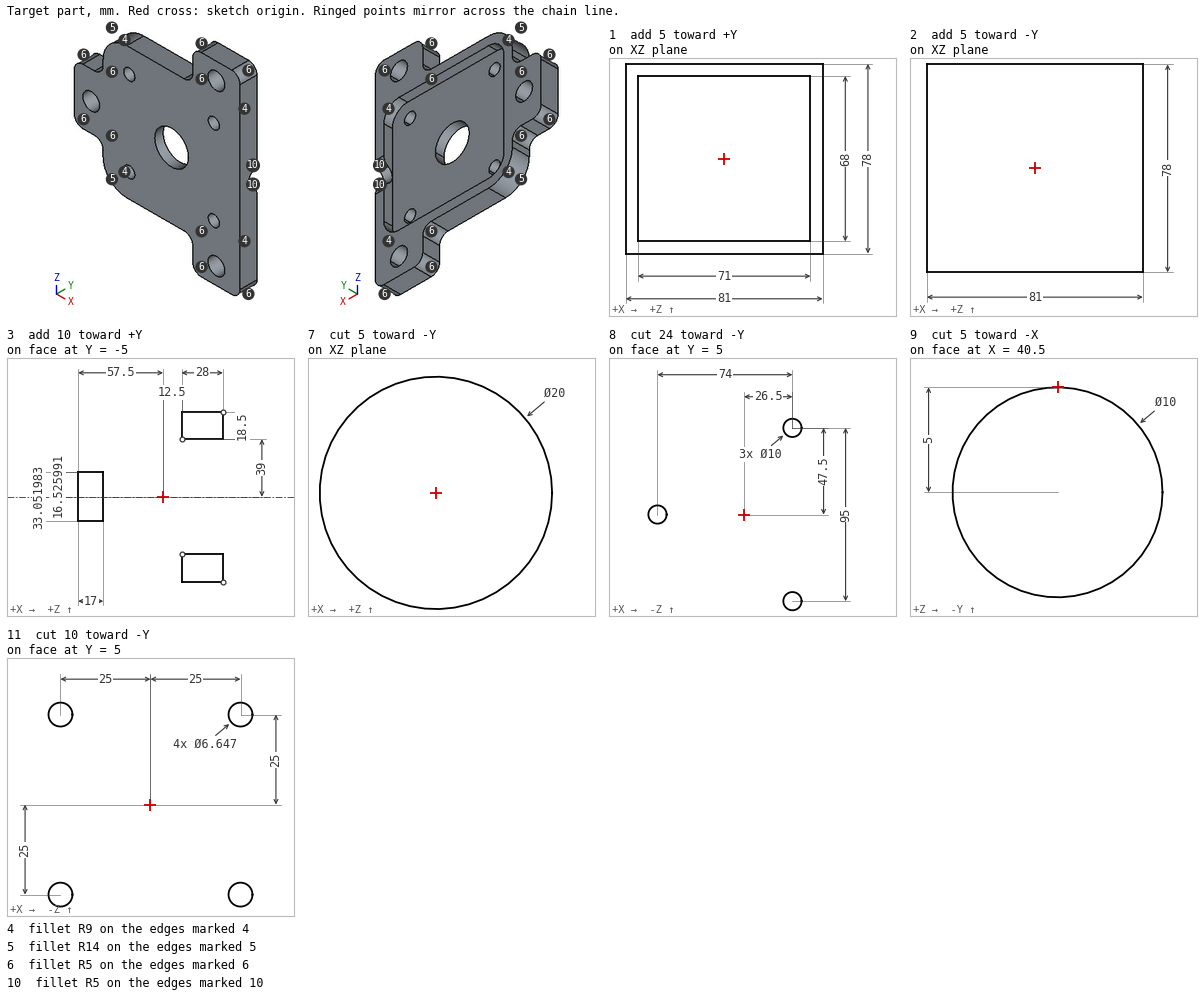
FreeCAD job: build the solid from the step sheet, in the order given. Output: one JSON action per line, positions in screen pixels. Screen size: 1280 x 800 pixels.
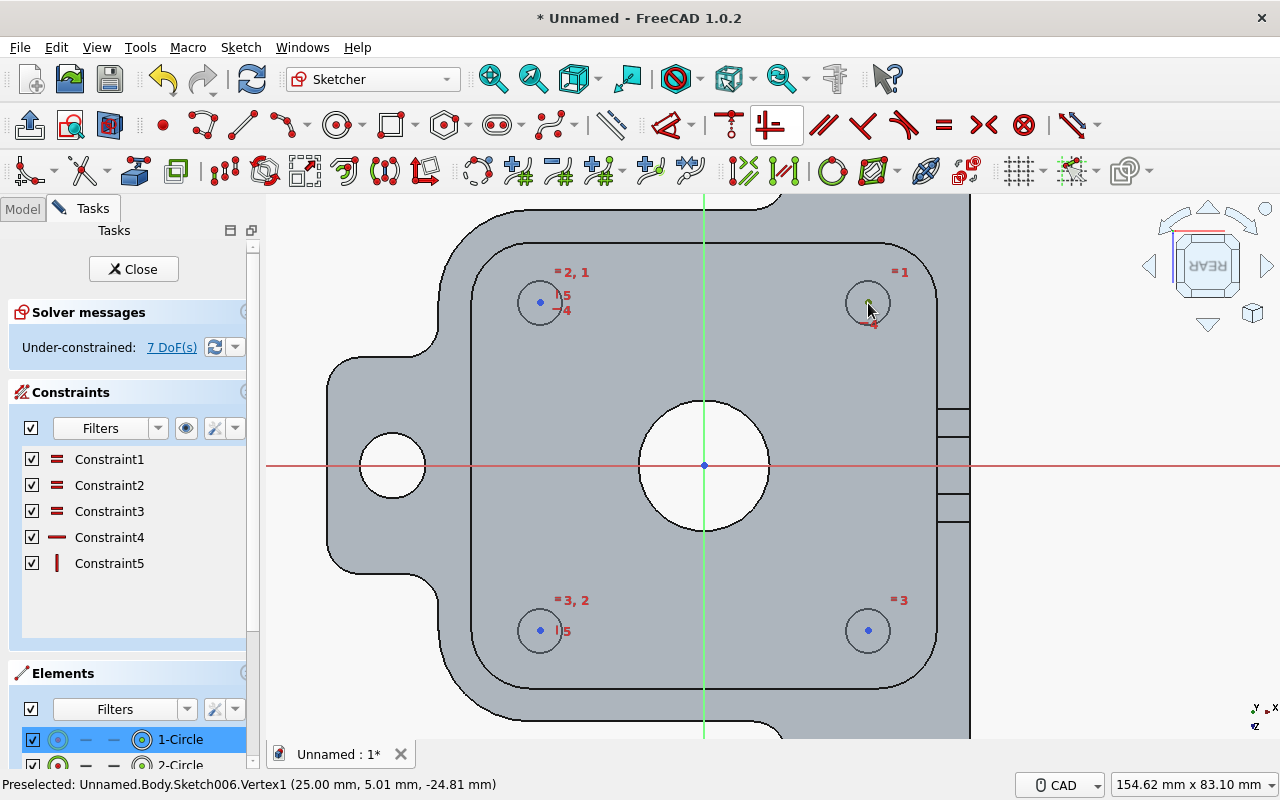
{"action": "left_click", "coordinate": [868, 631]}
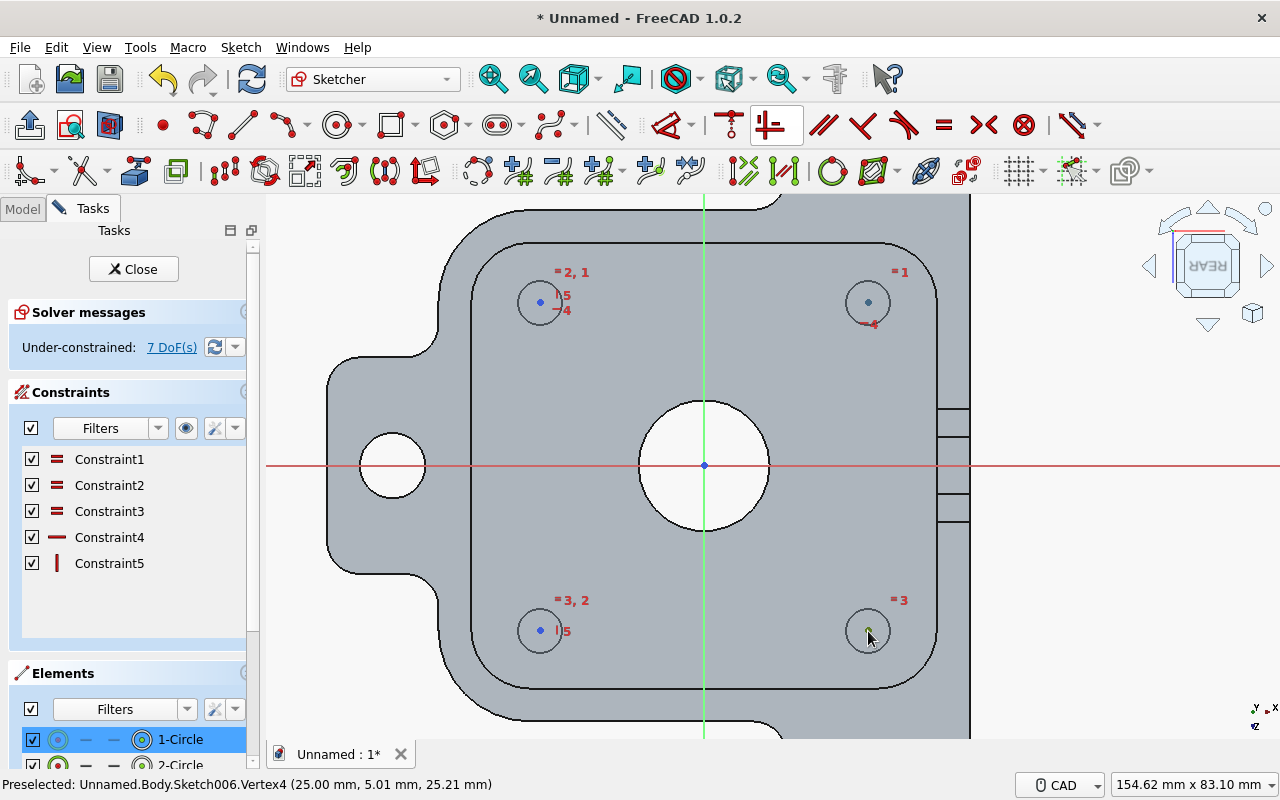
{"action": "left_click", "coordinate": [798, 126]}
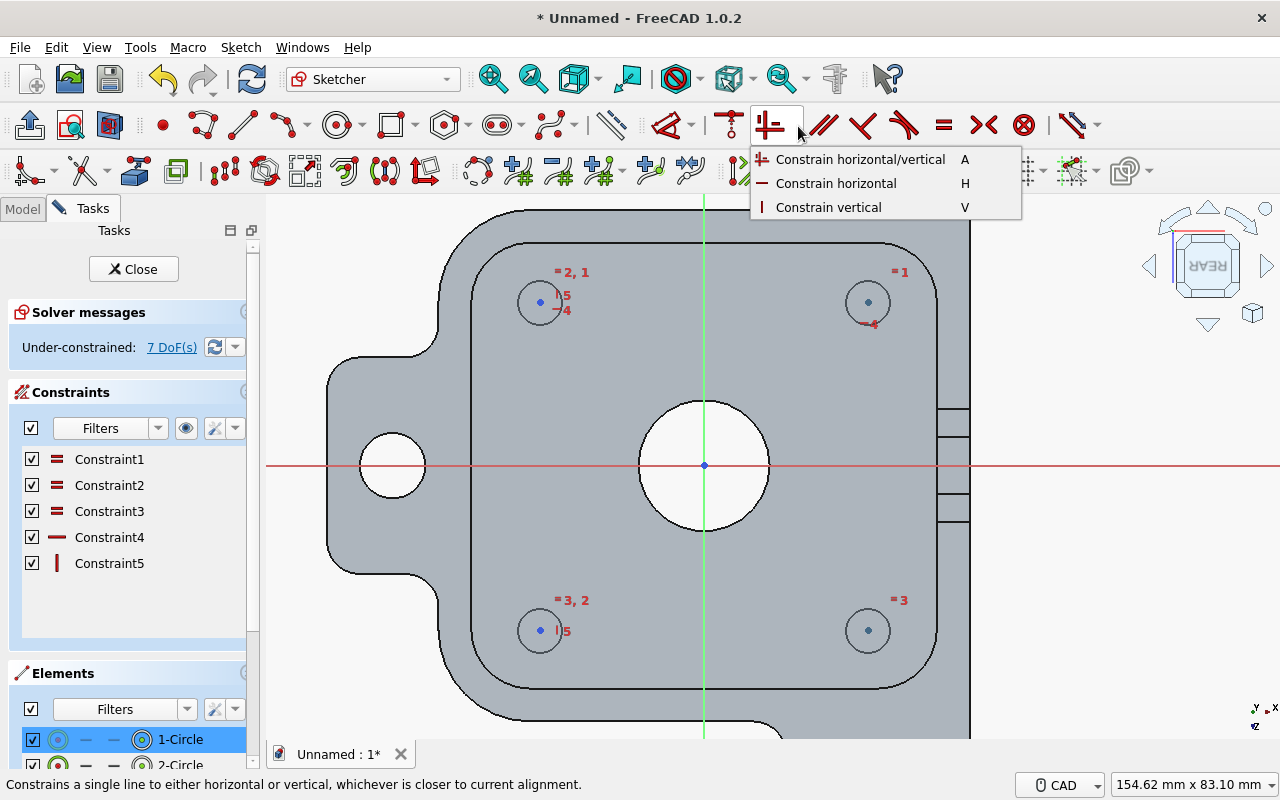
{"action": "left_click", "coordinate": [886, 207]}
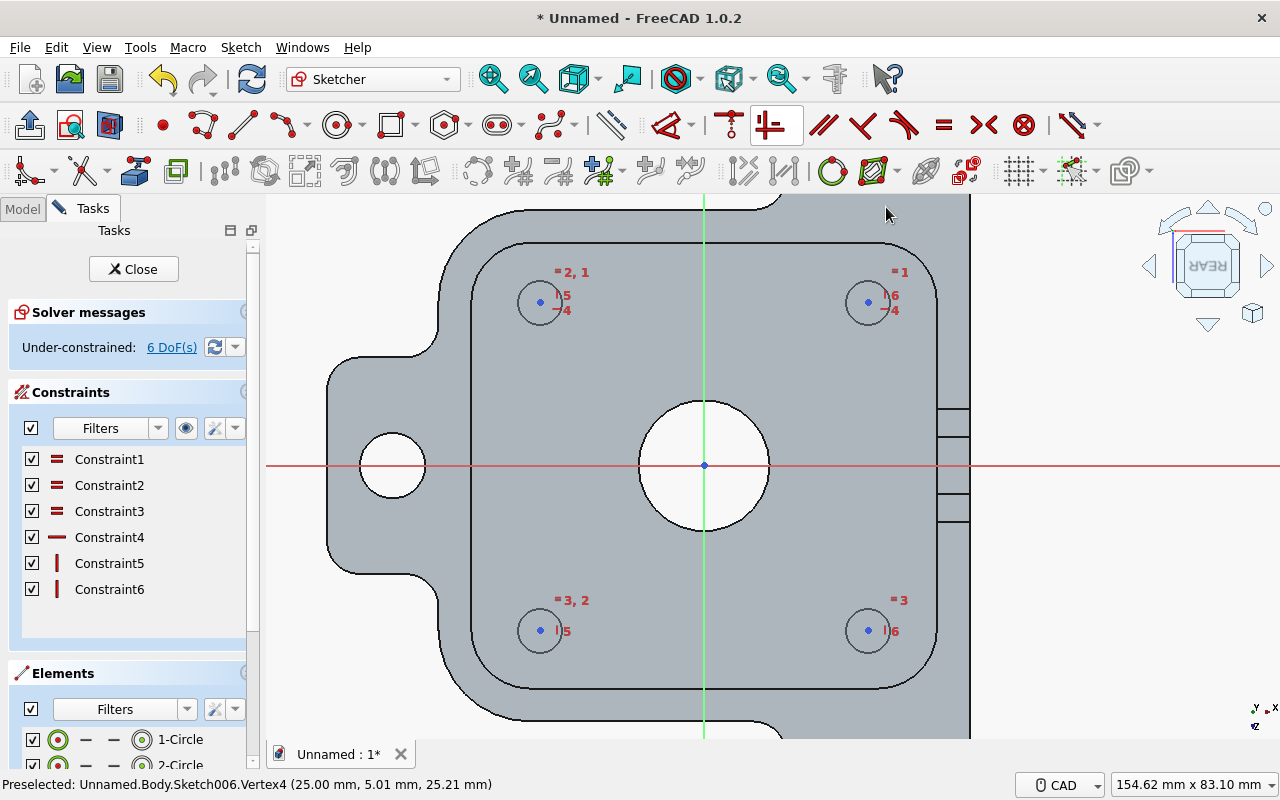
{"action": "left_click", "coordinate": [540, 631]}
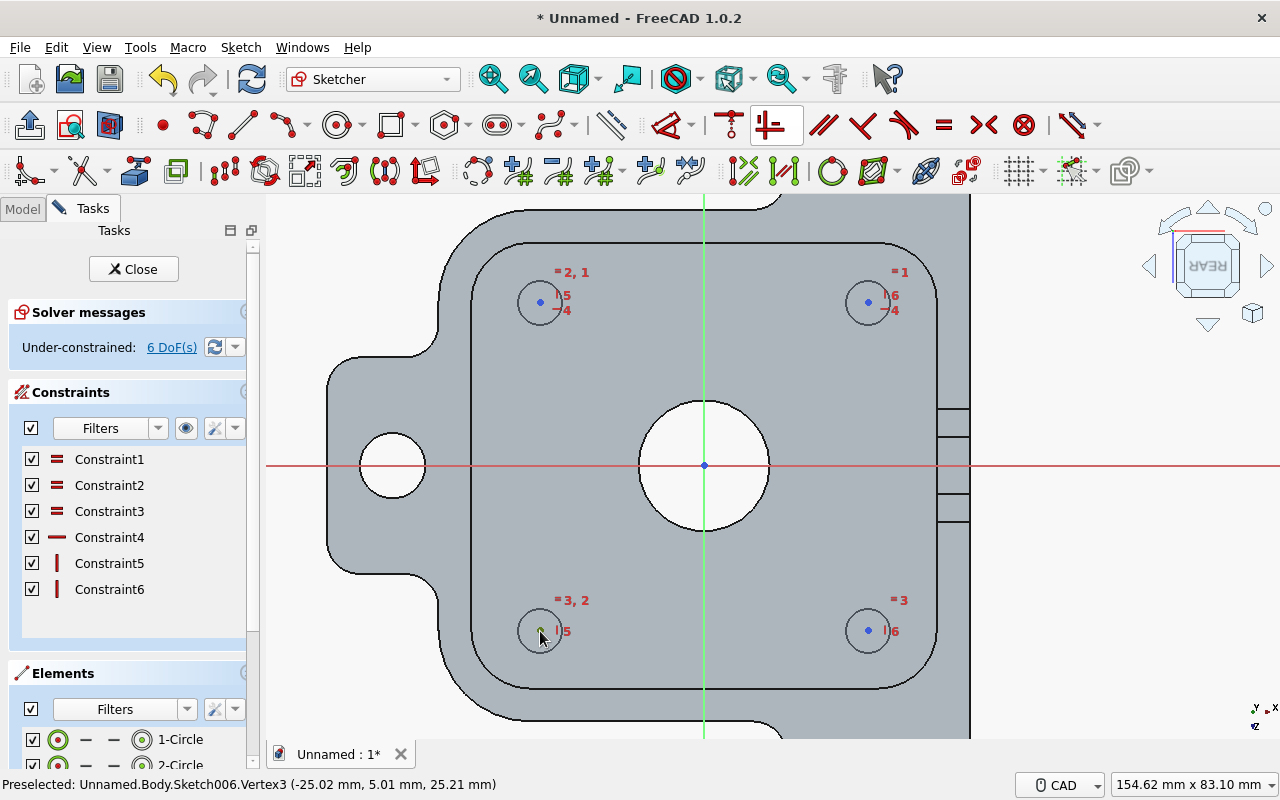
{"action": "left_click", "coordinate": [868, 631]}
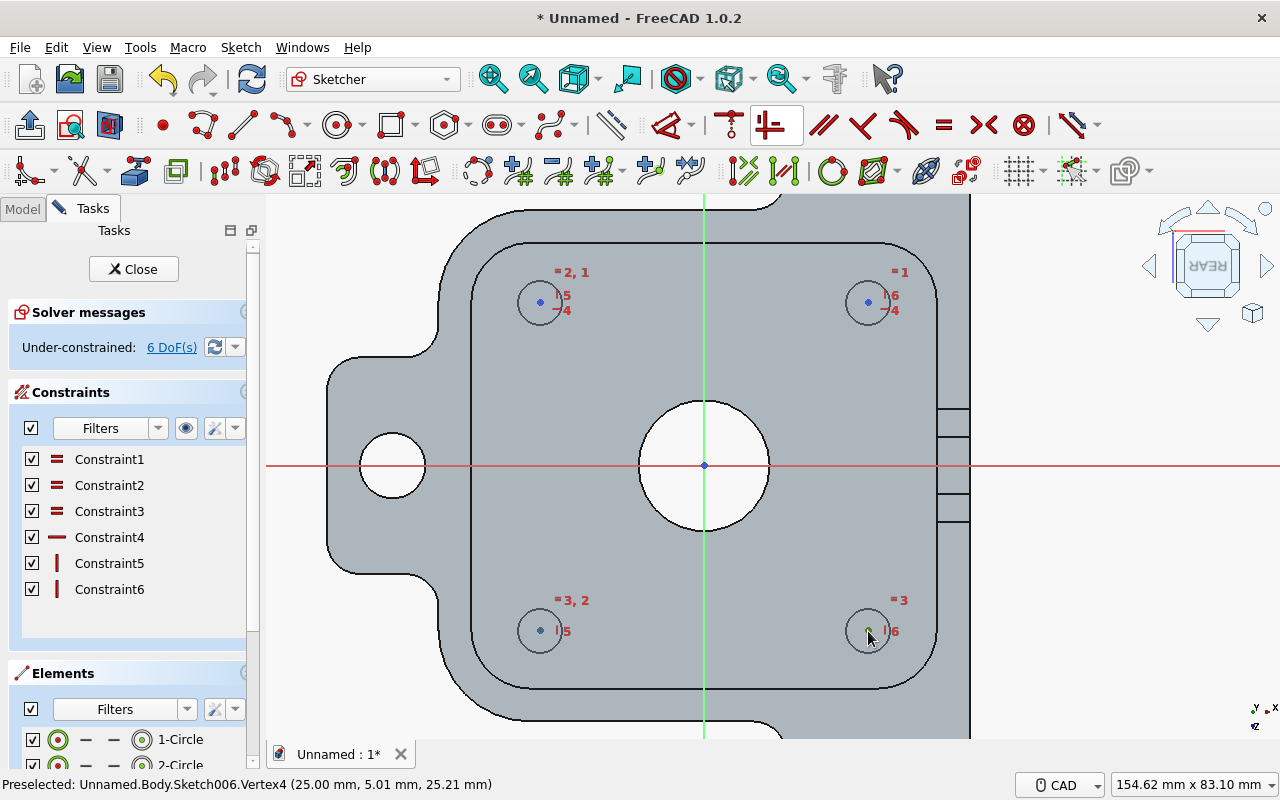
{"action": "key", "text": "h"}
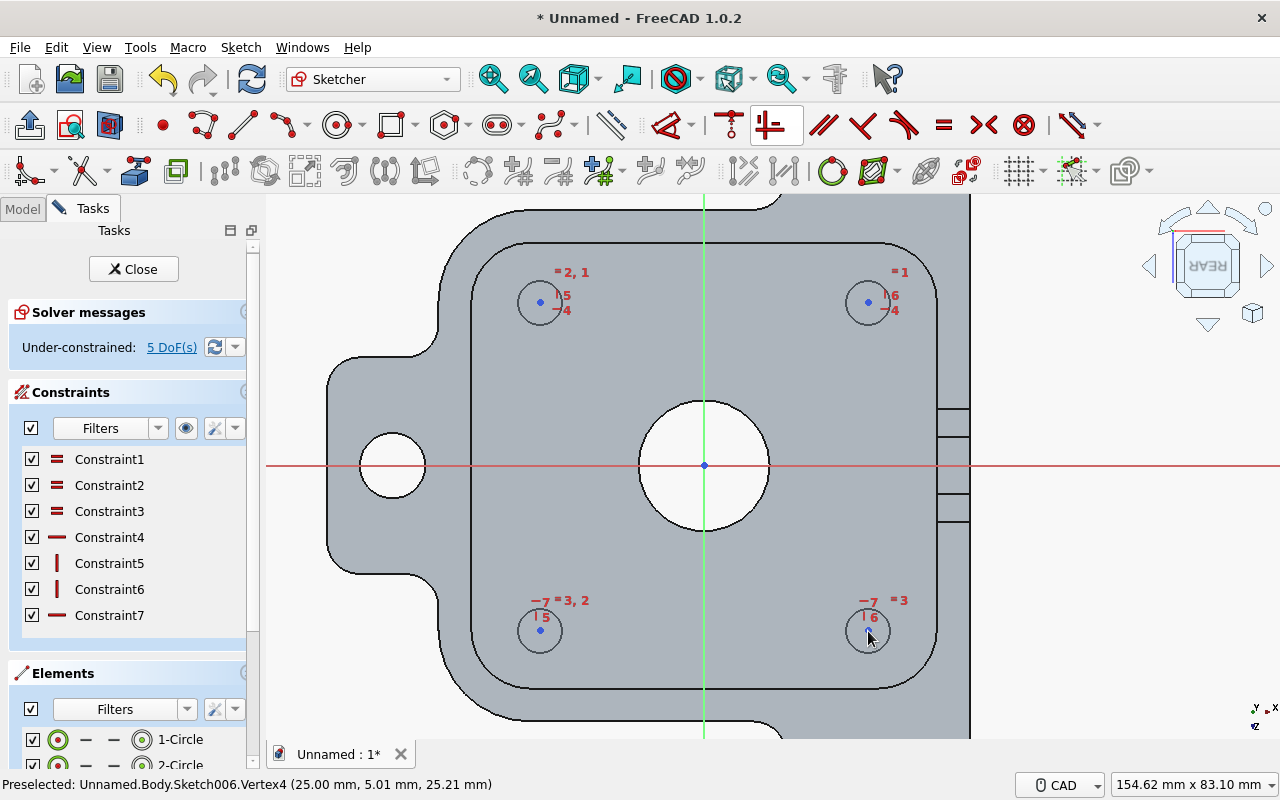
{"action": "key", "text": "d"}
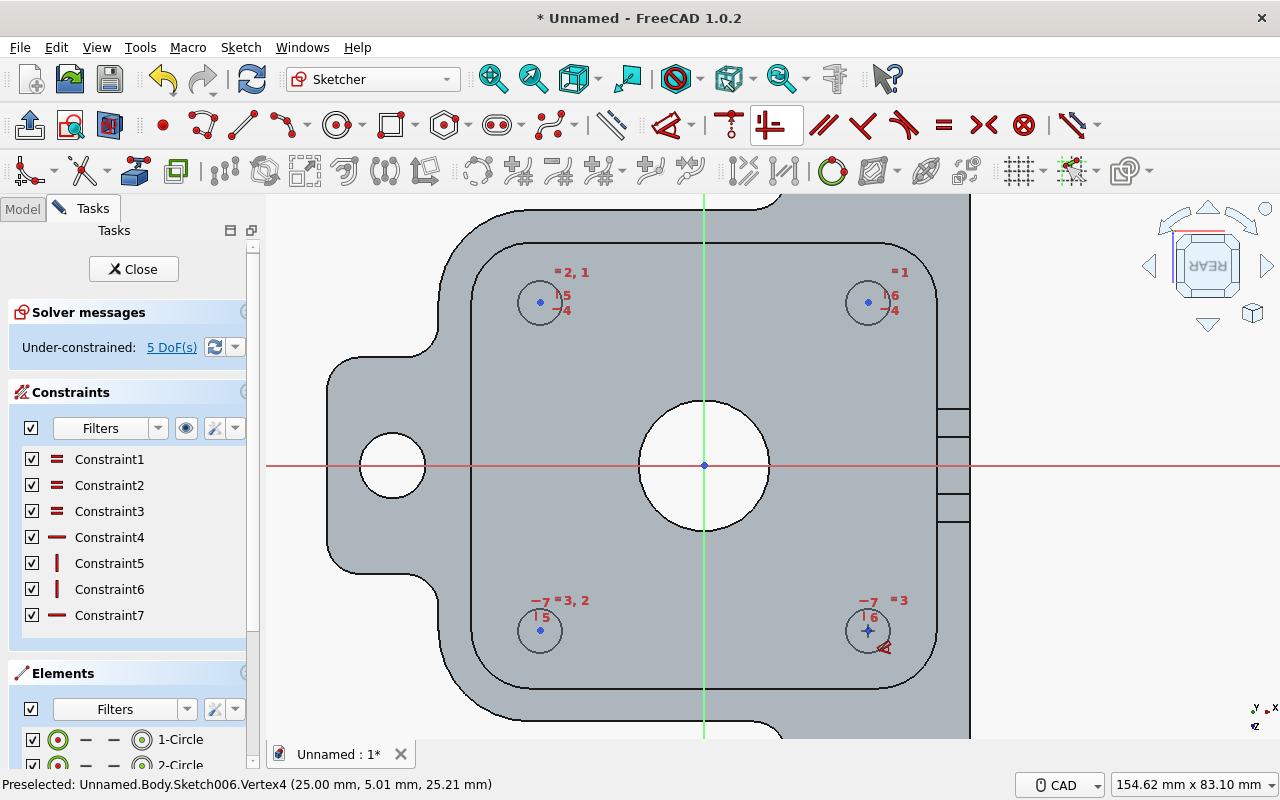
{"action": "left_click", "coordinate": [883, 287]}
{"action": "left_click", "coordinate": [905, 264]}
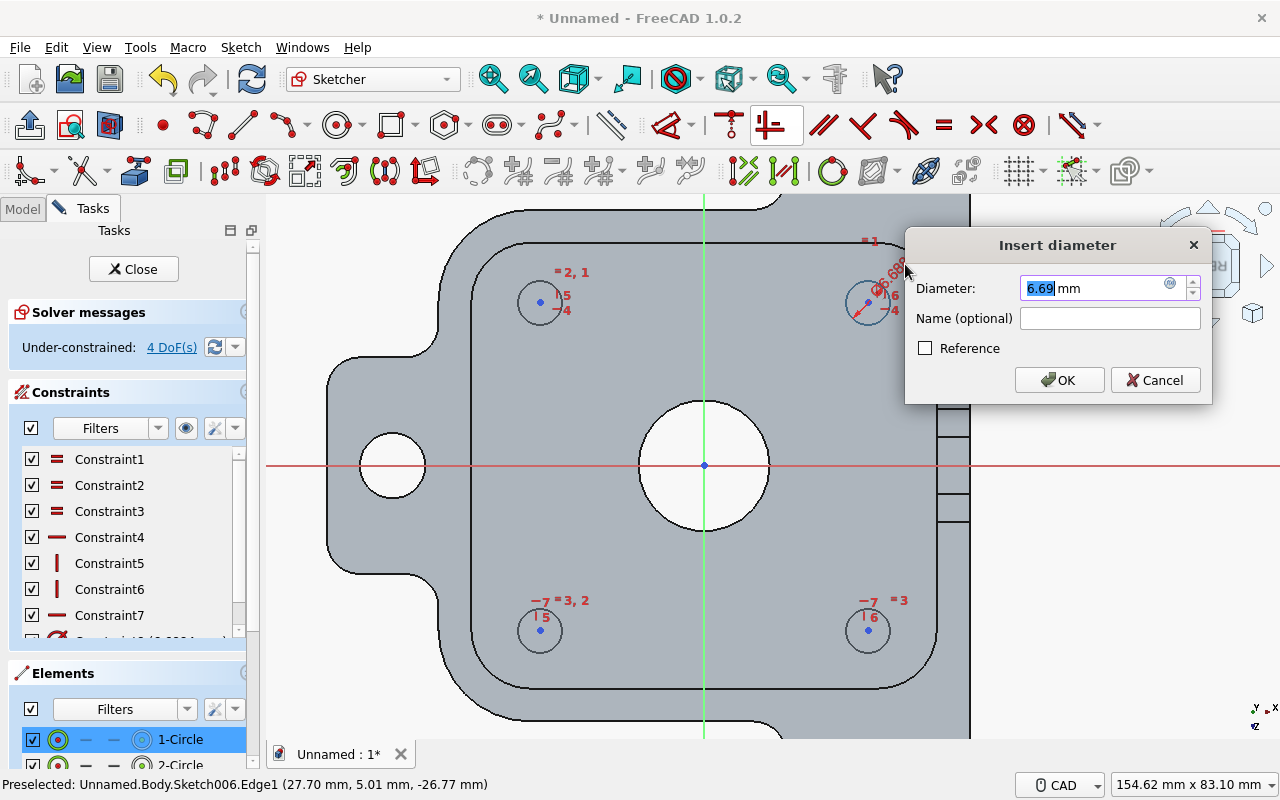
{"action": "type", "text": "6.647"}
{"action": "key", "text": "Return"}